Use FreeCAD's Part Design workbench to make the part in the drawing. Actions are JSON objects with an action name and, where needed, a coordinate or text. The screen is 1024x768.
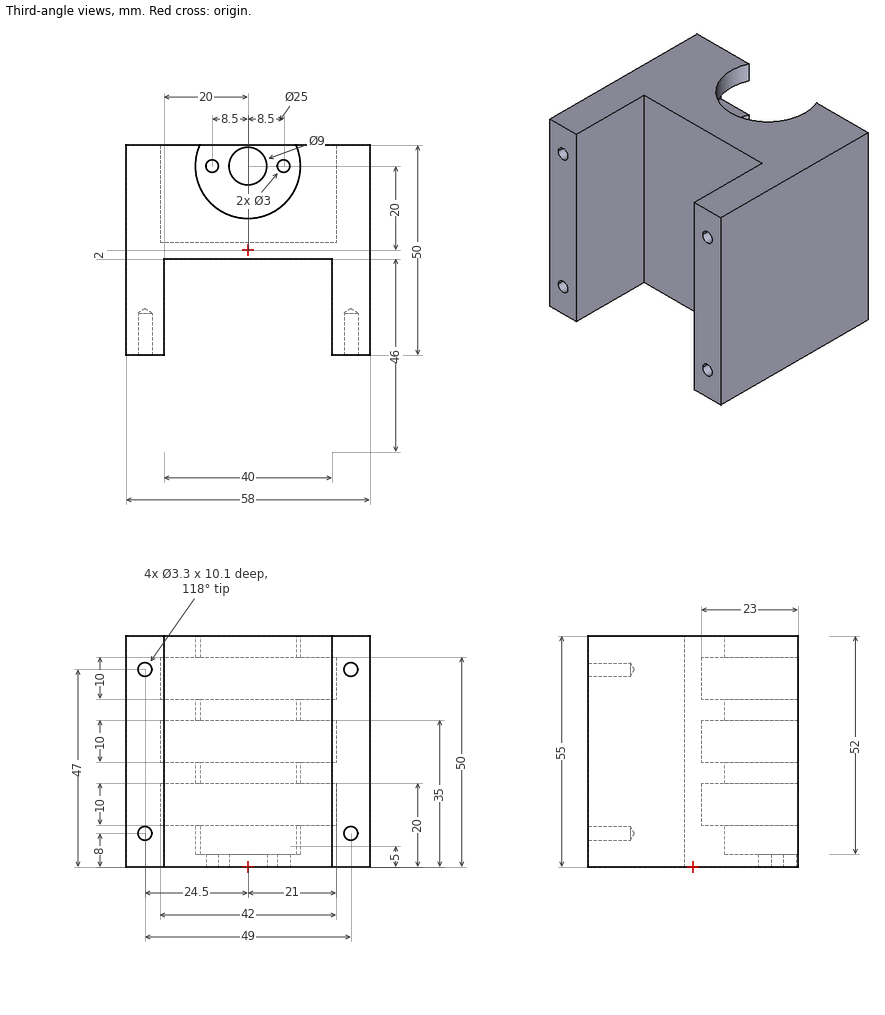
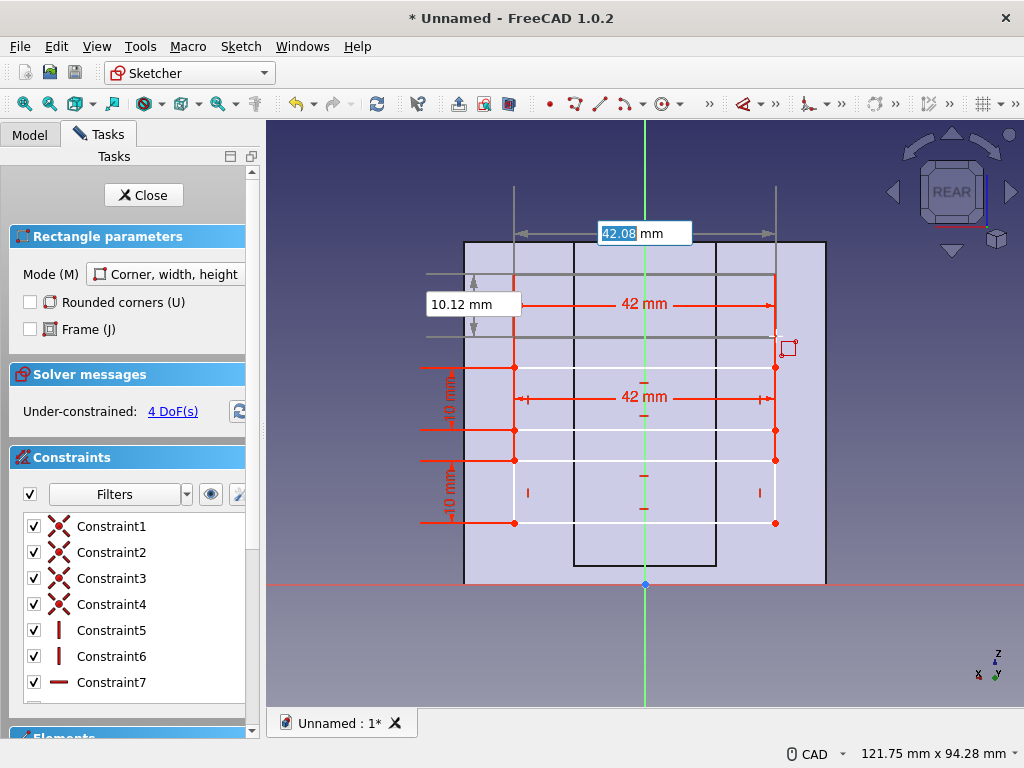
{"action": "type", "text": "42"}
{"action": "key", "text": "Tab"}
{"action": "type", "text": "10"}
{"action": "key", "text": "Return"}
{"action": "key", "text": "Escape"}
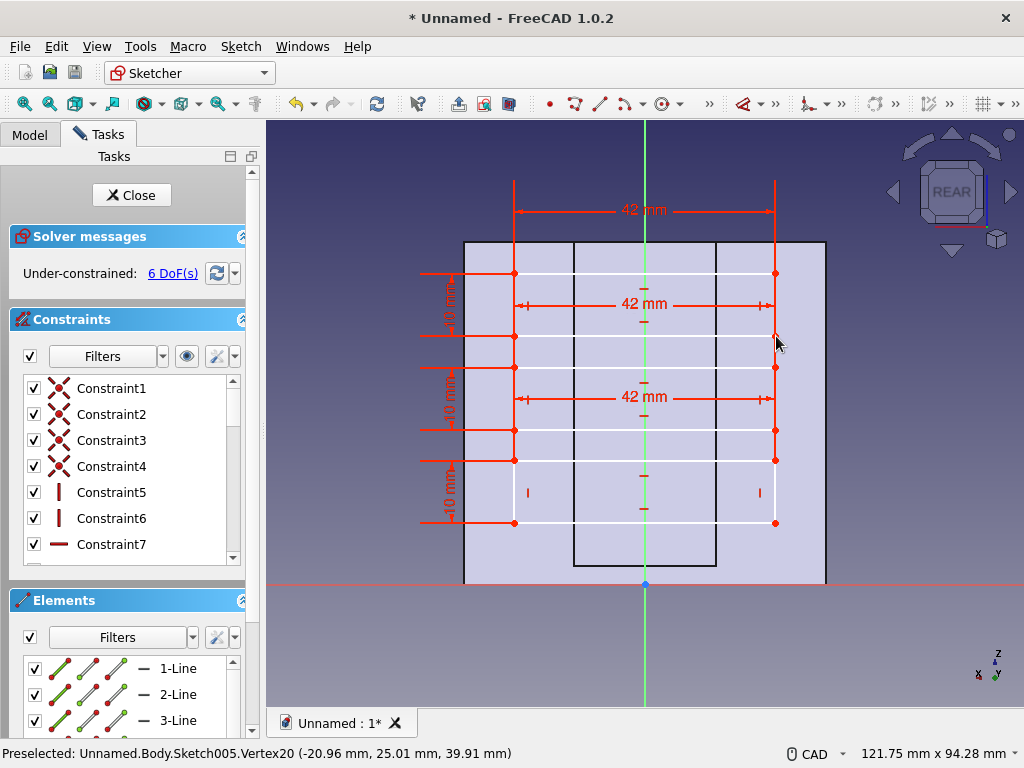
{"action": "left_click", "coordinate": [742, 104]}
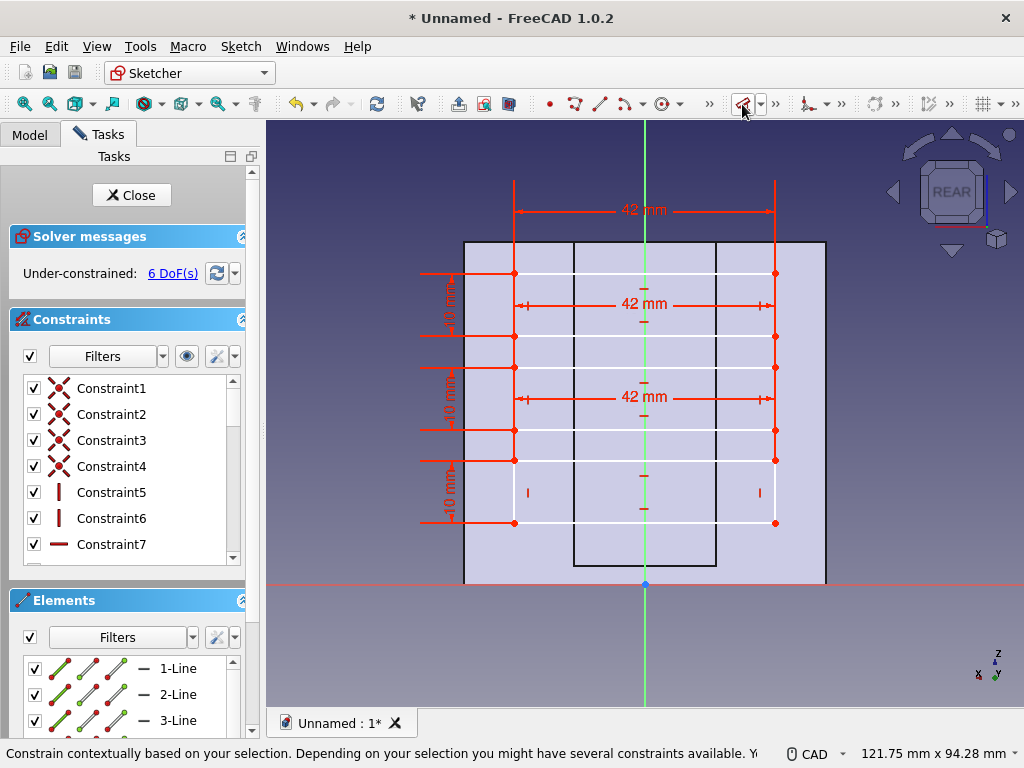
{"action": "left_click", "coordinate": [514, 461]}
{"action": "left_click", "coordinate": [580, 619]}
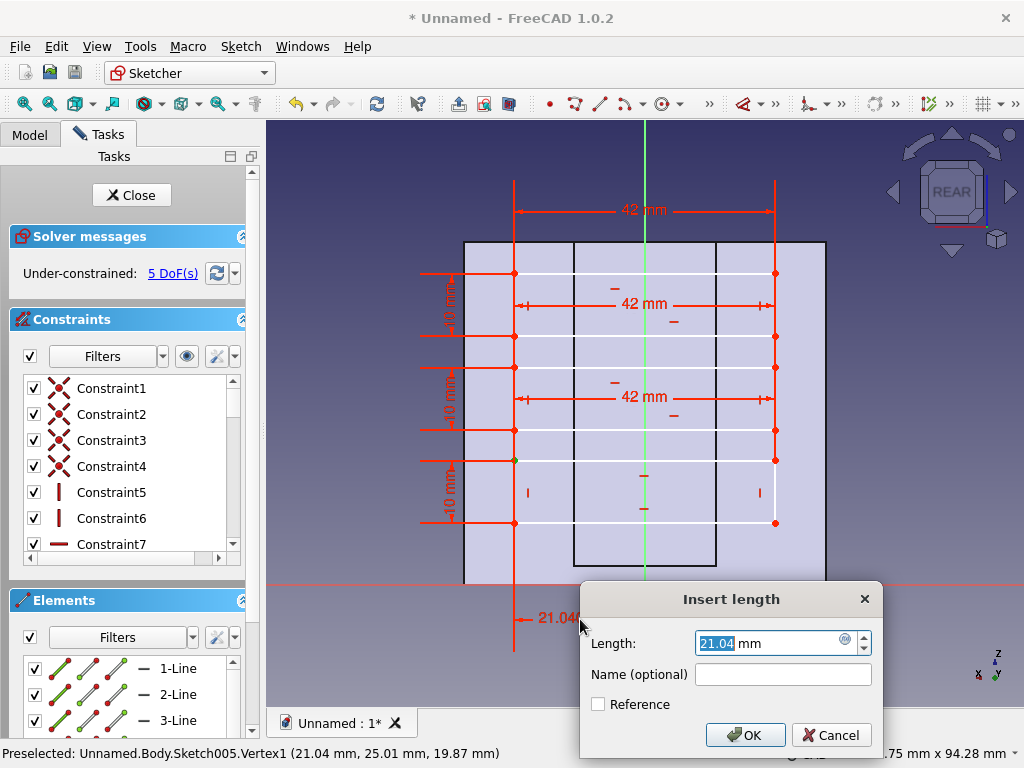
{"action": "type", "text": "21"}
{"action": "key", "text": "Return"}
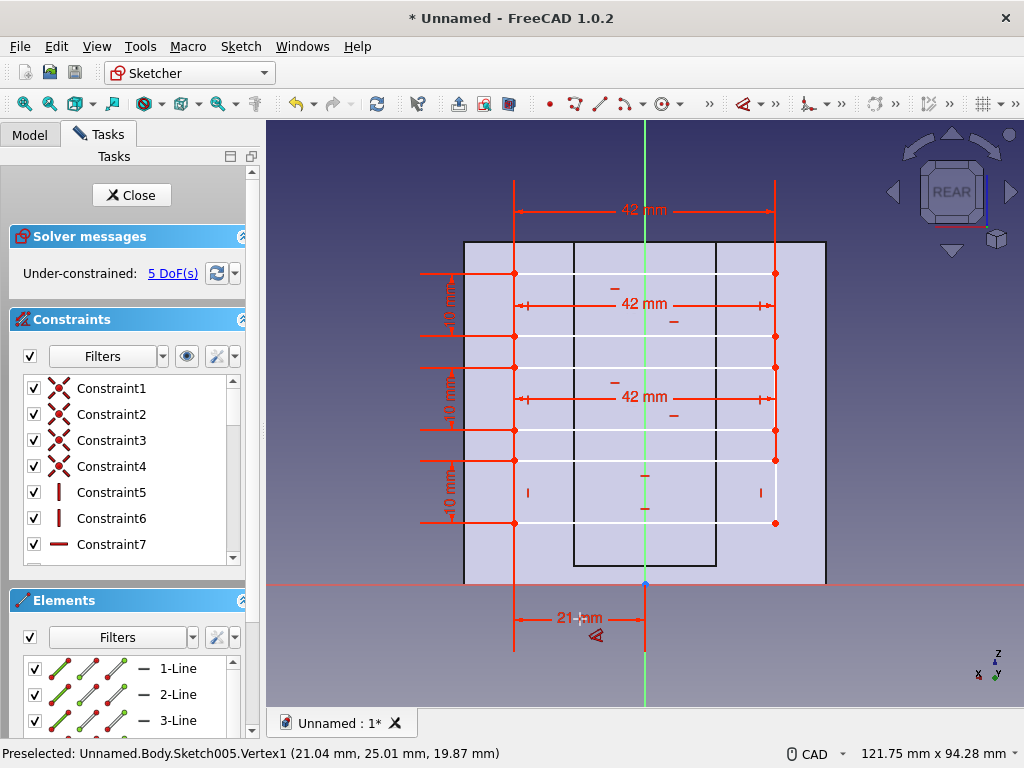
{"action": "left_click", "coordinate": [514, 461]}
{"action": "left_click", "coordinate": [480, 523]}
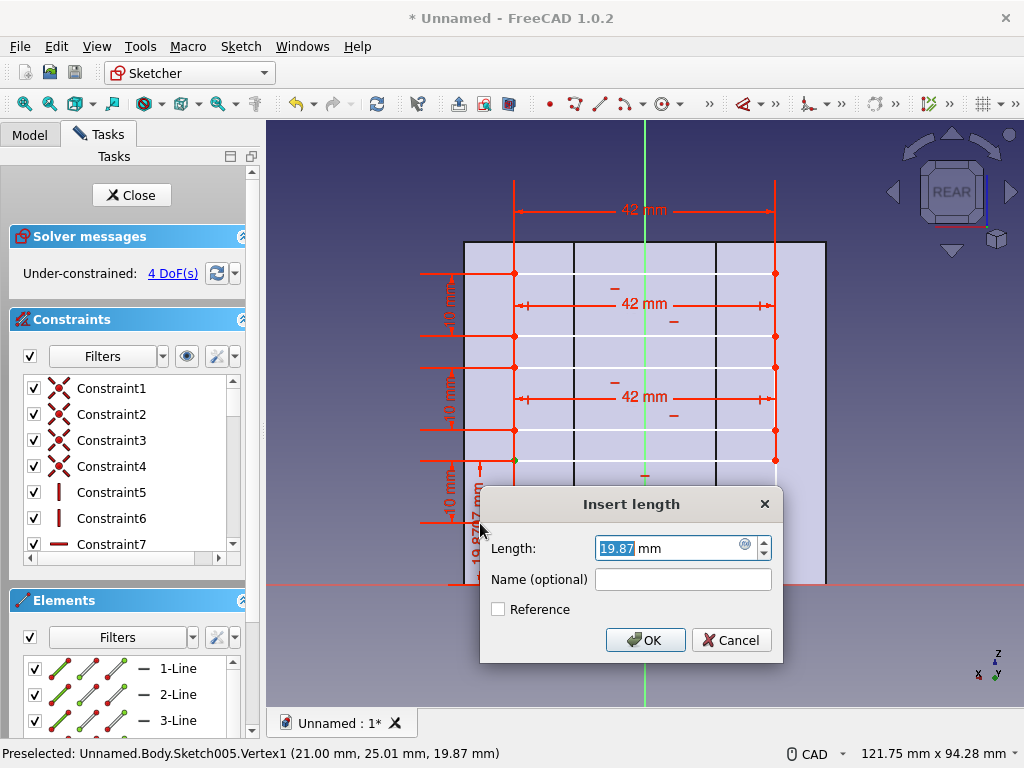
{"action": "type", "text": "20"}
{"action": "key", "text": "Return"}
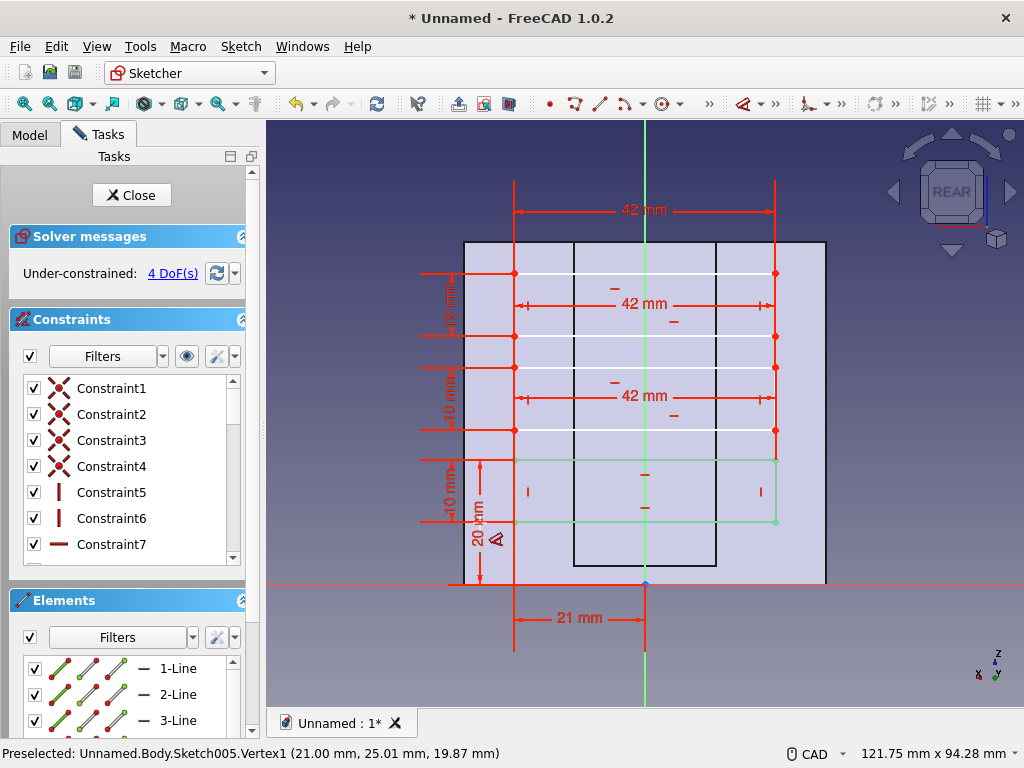
{"action": "left_click", "coordinate": [514, 368]}
{"action": "left_click", "coordinate": [580, 643]}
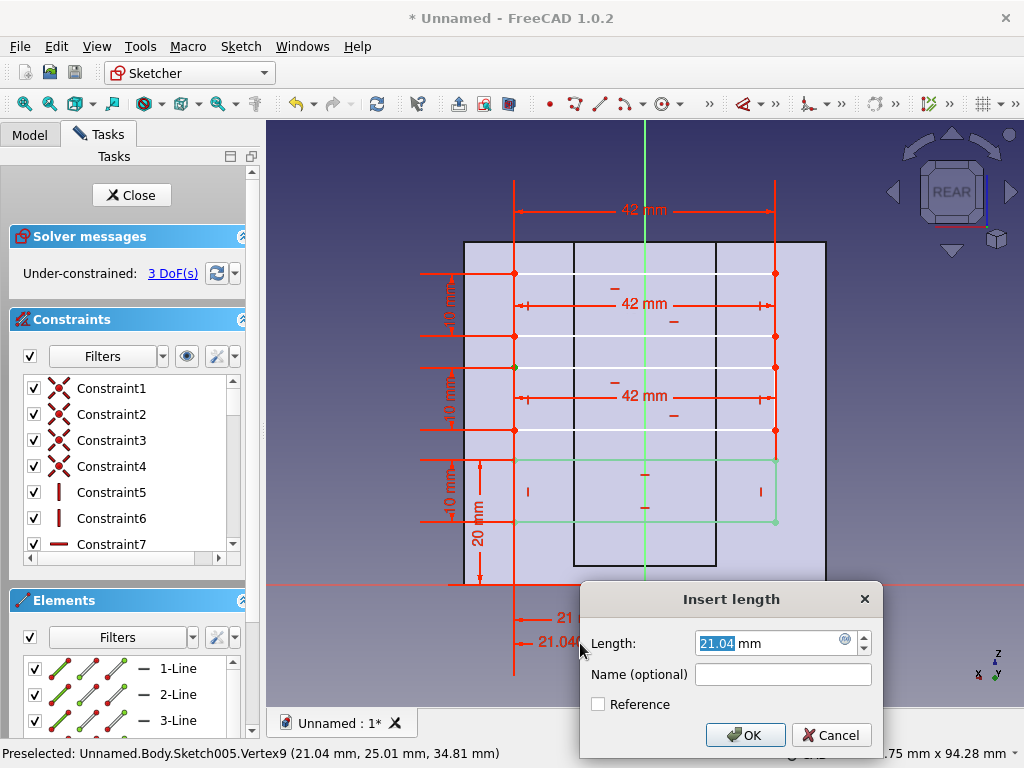
{"action": "type", "text": "21"}
{"action": "key", "text": "Return"}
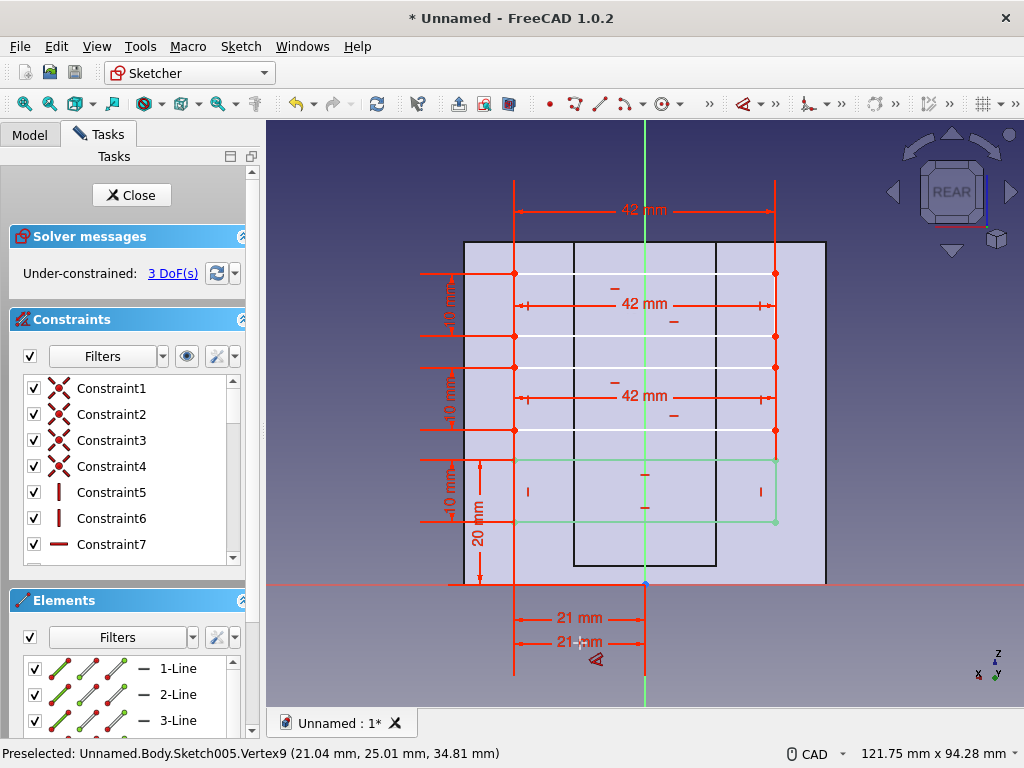
{"action": "left_click", "coordinate": [514, 368]}
{"action": "left_click", "coordinate": [480, 476]}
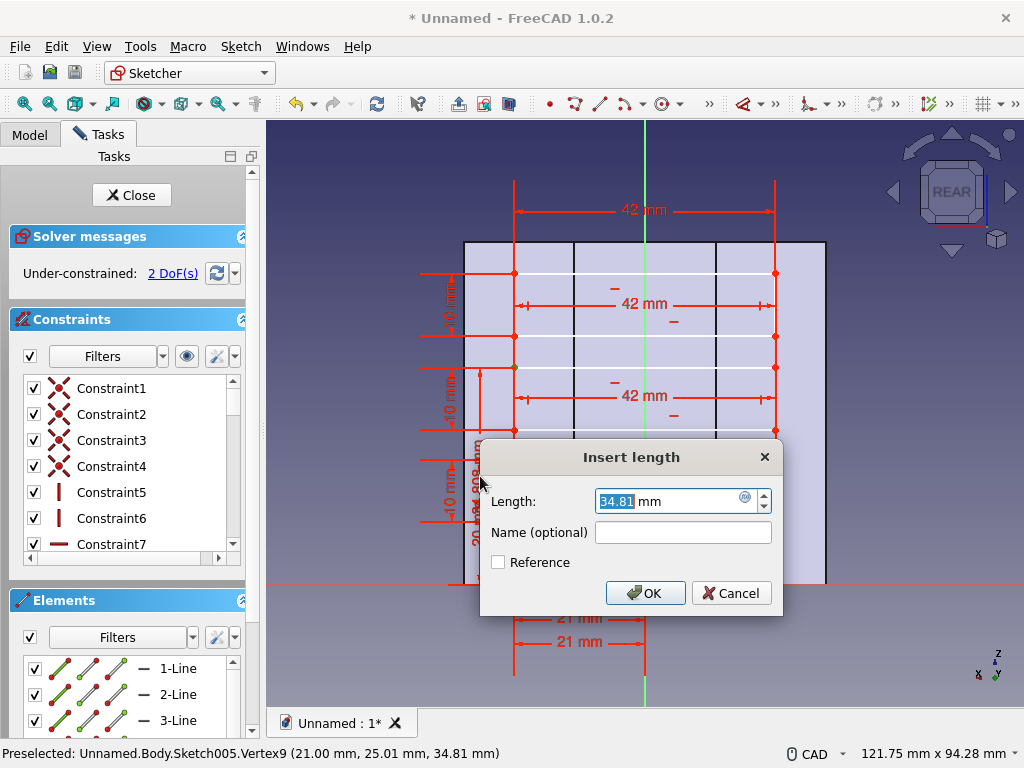
{"action": "type", "text": "35"}
{"action": "key", "text": "Return"}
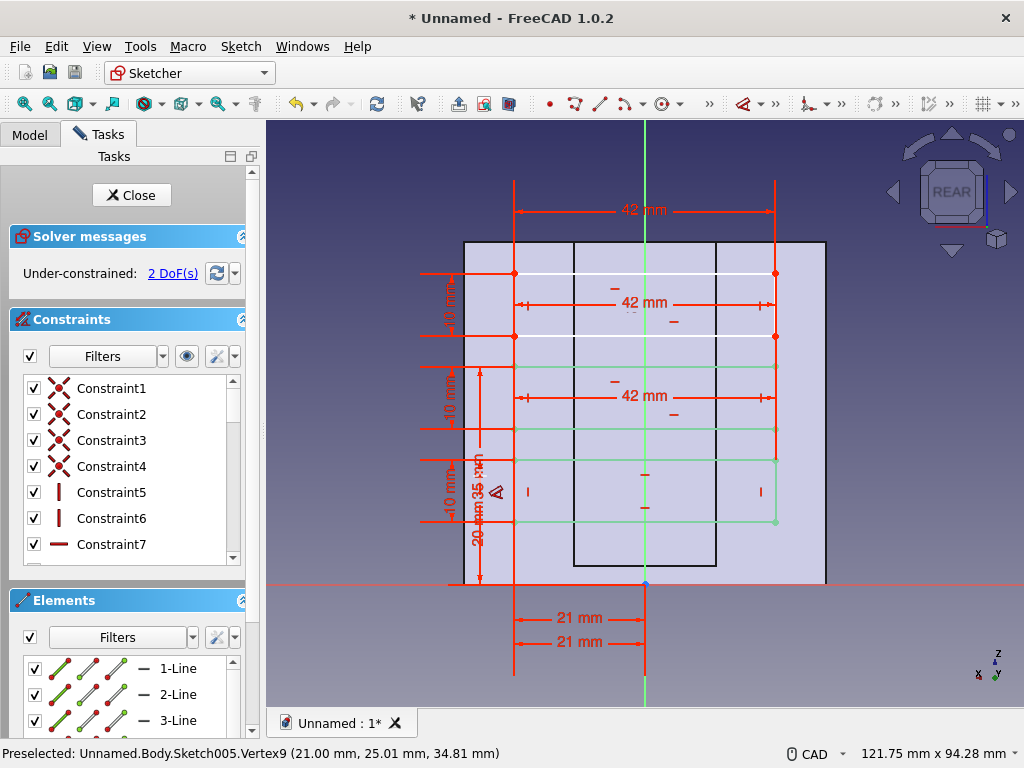
{"action": "left_click", "coordinate": [514, 274]}
{"action": "left_click", "coordinate": [580, 240]}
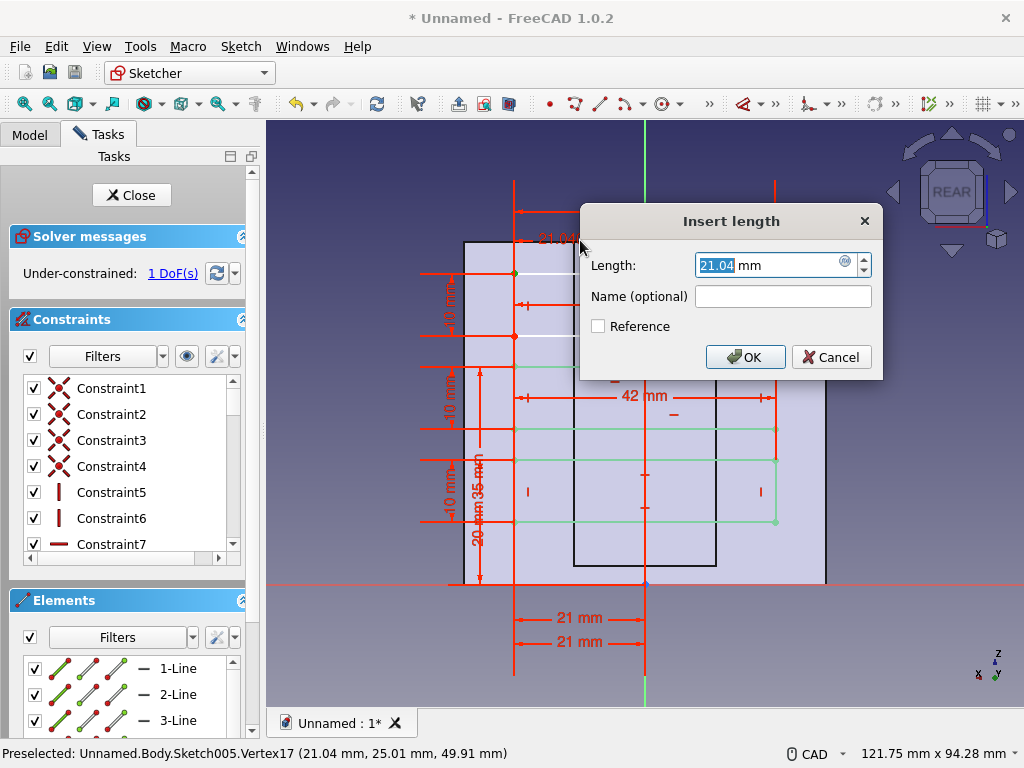
{"action": "type", "text": "21"}
{"action": "key", "text": "Return"}